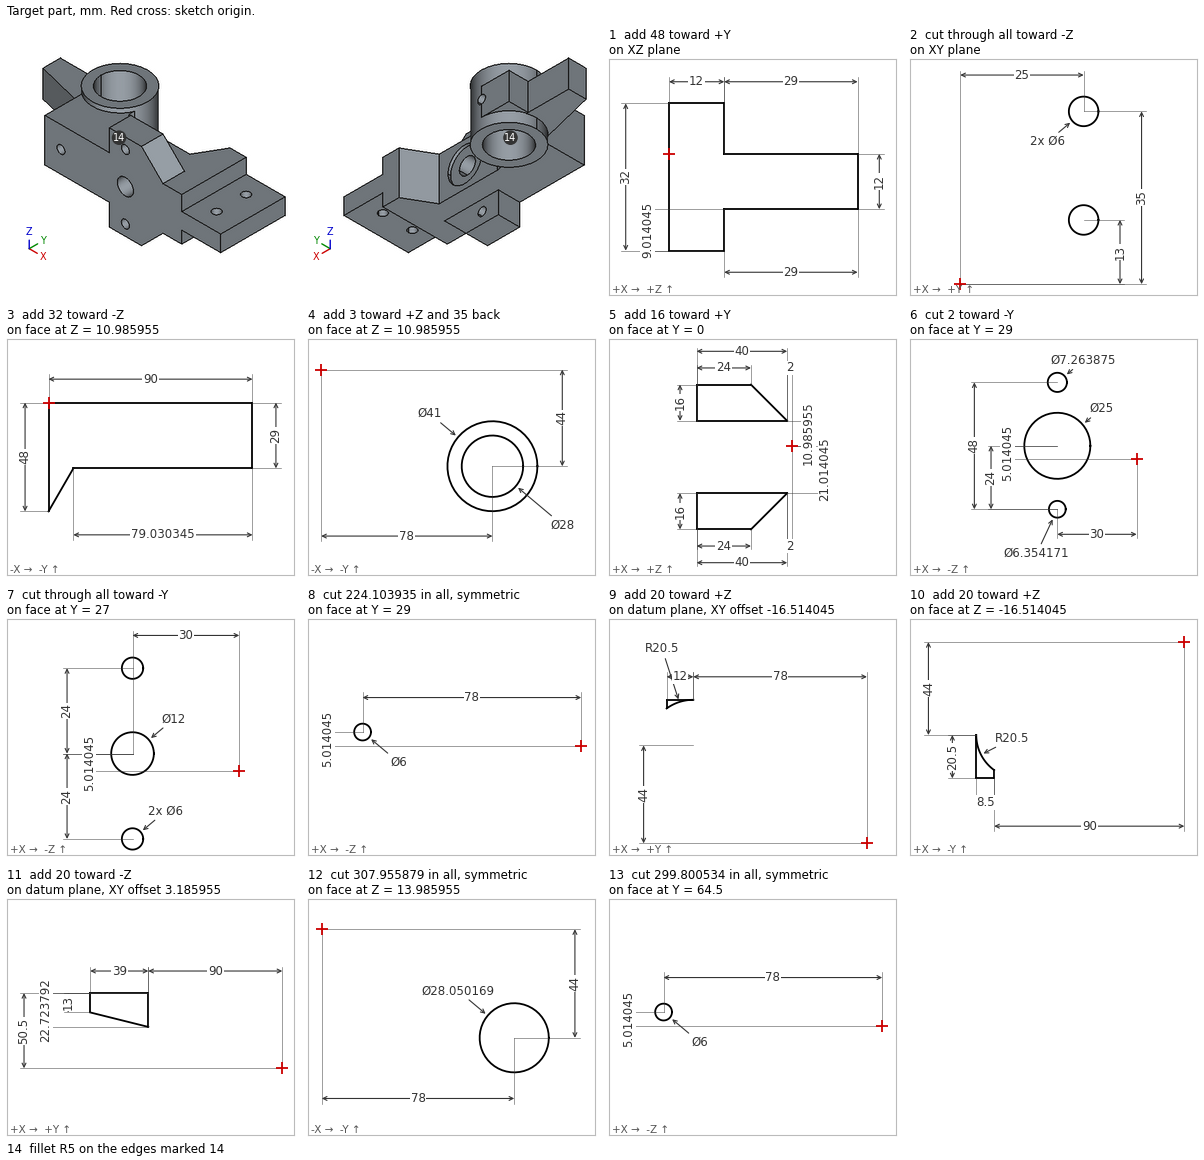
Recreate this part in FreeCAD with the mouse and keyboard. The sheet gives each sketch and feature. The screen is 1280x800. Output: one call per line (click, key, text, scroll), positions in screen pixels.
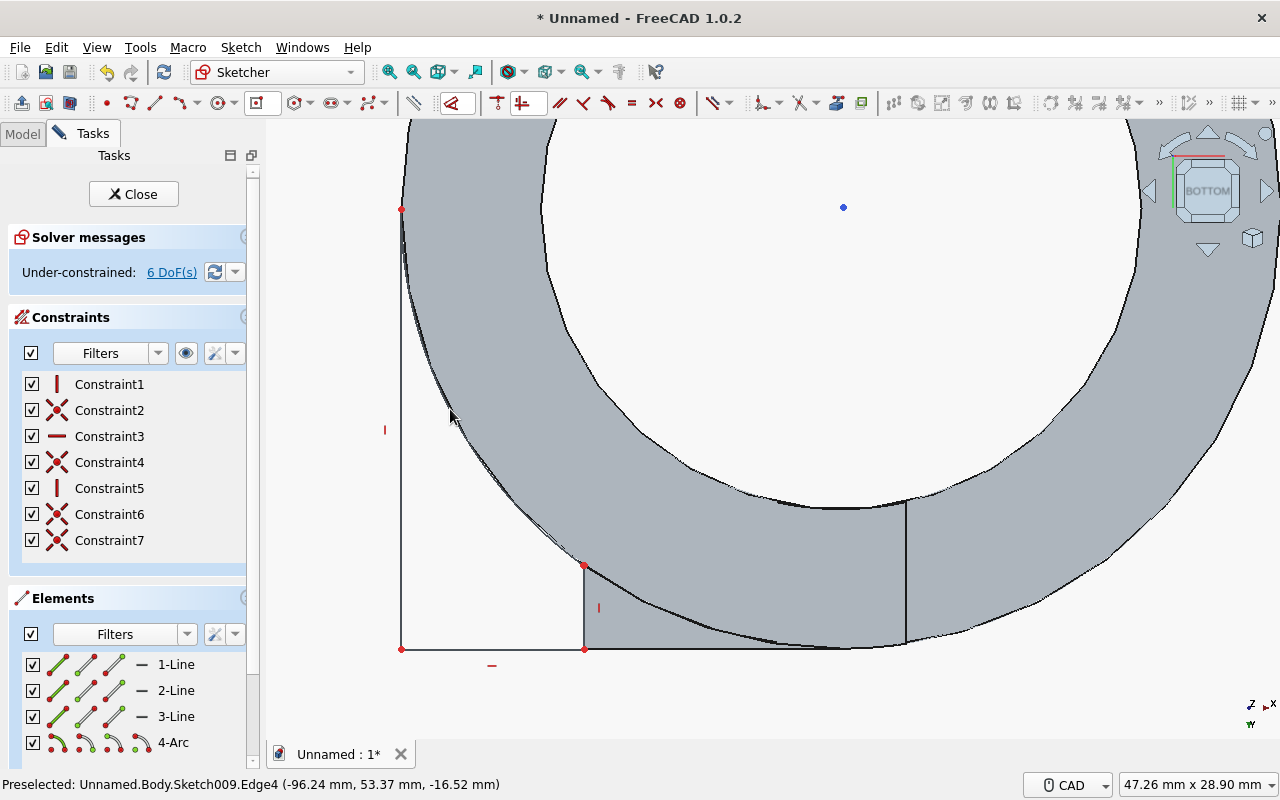
click(401, 518)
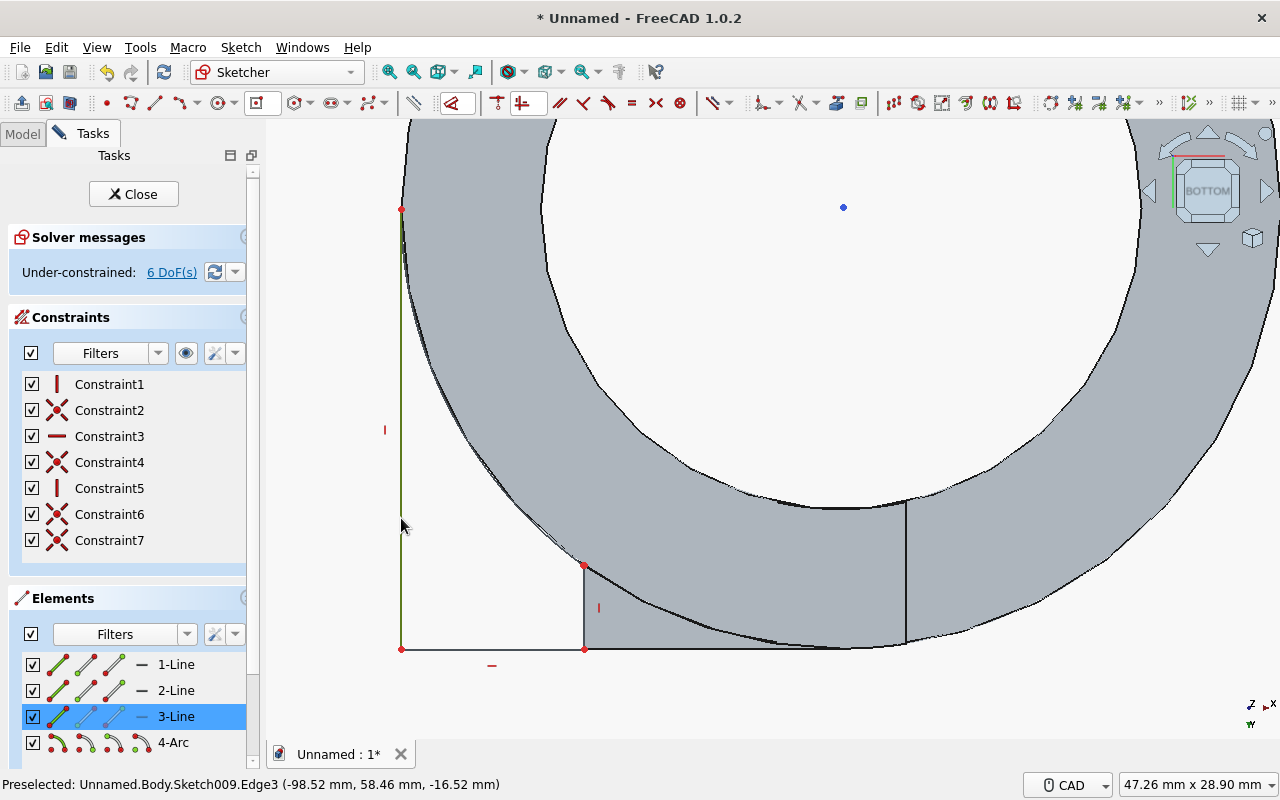
click(419, 333)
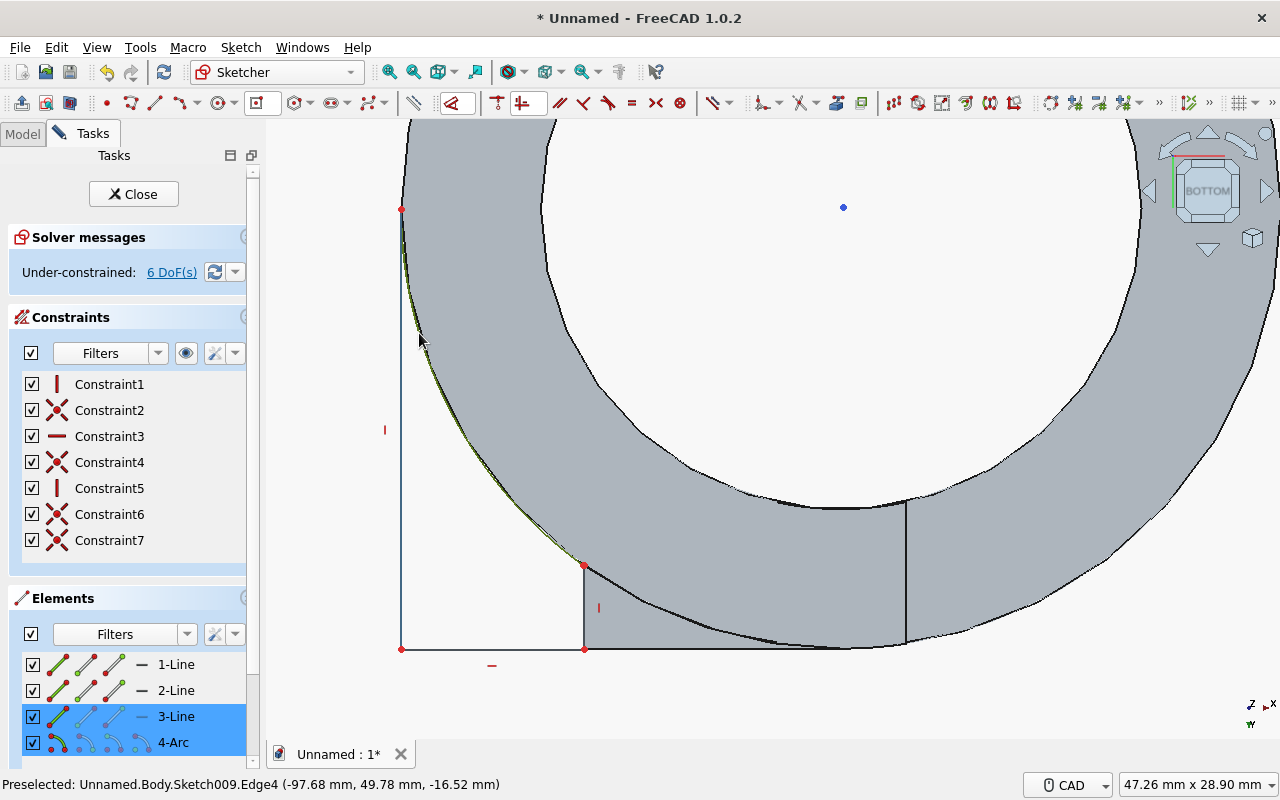
click(608, 104)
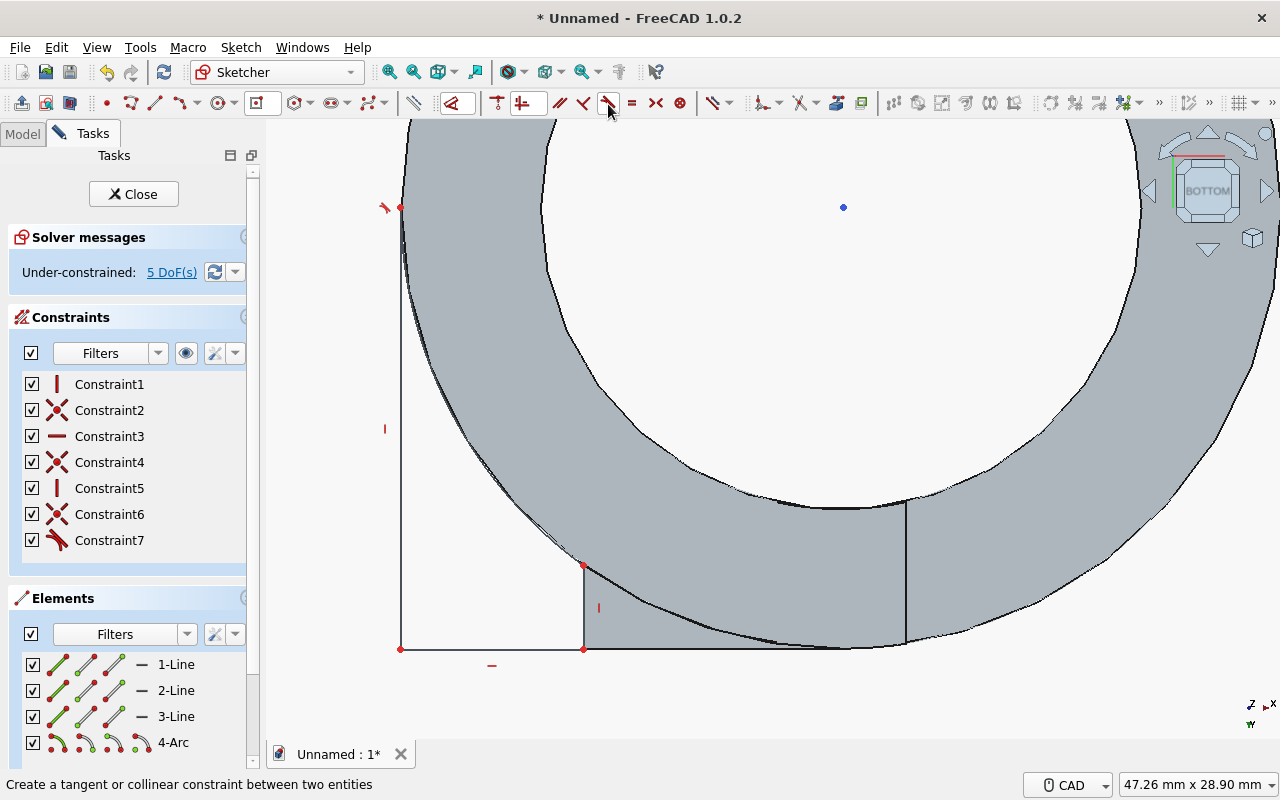
click(419, 331)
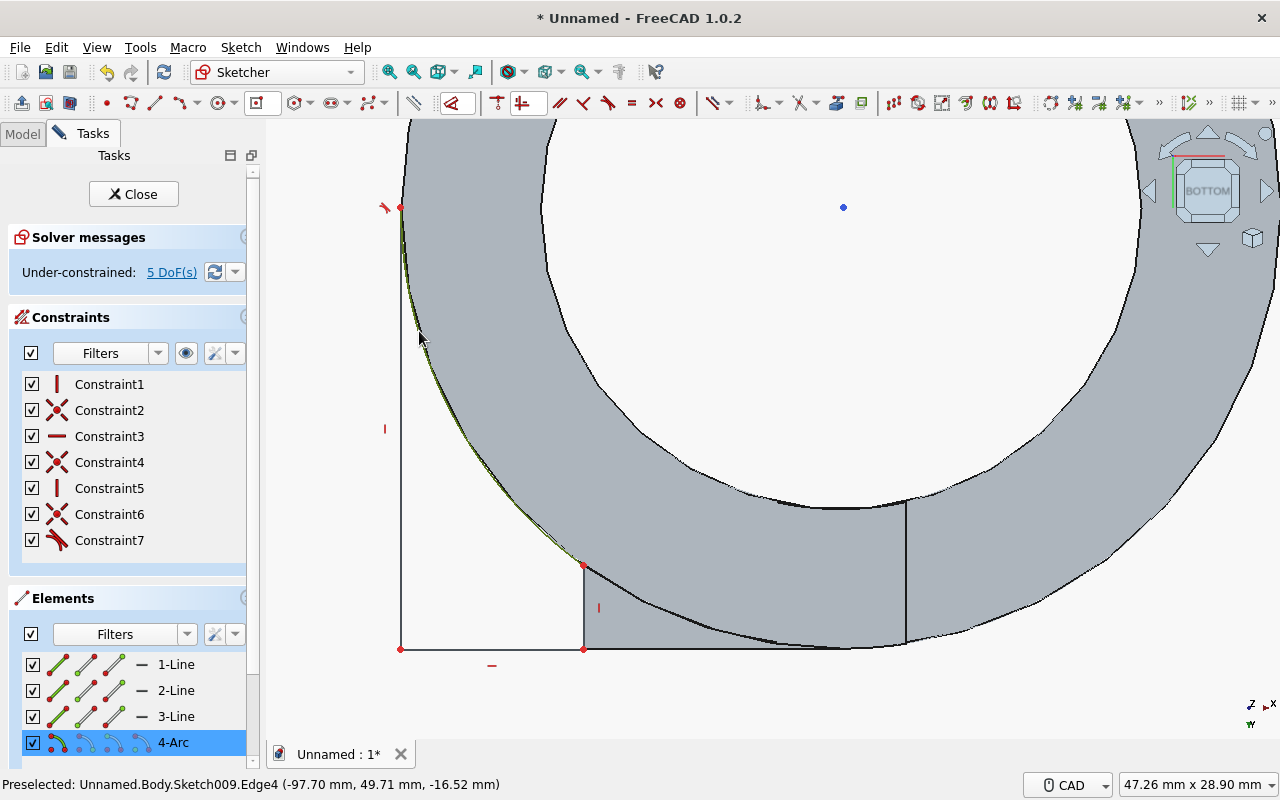
key(k)
key(r)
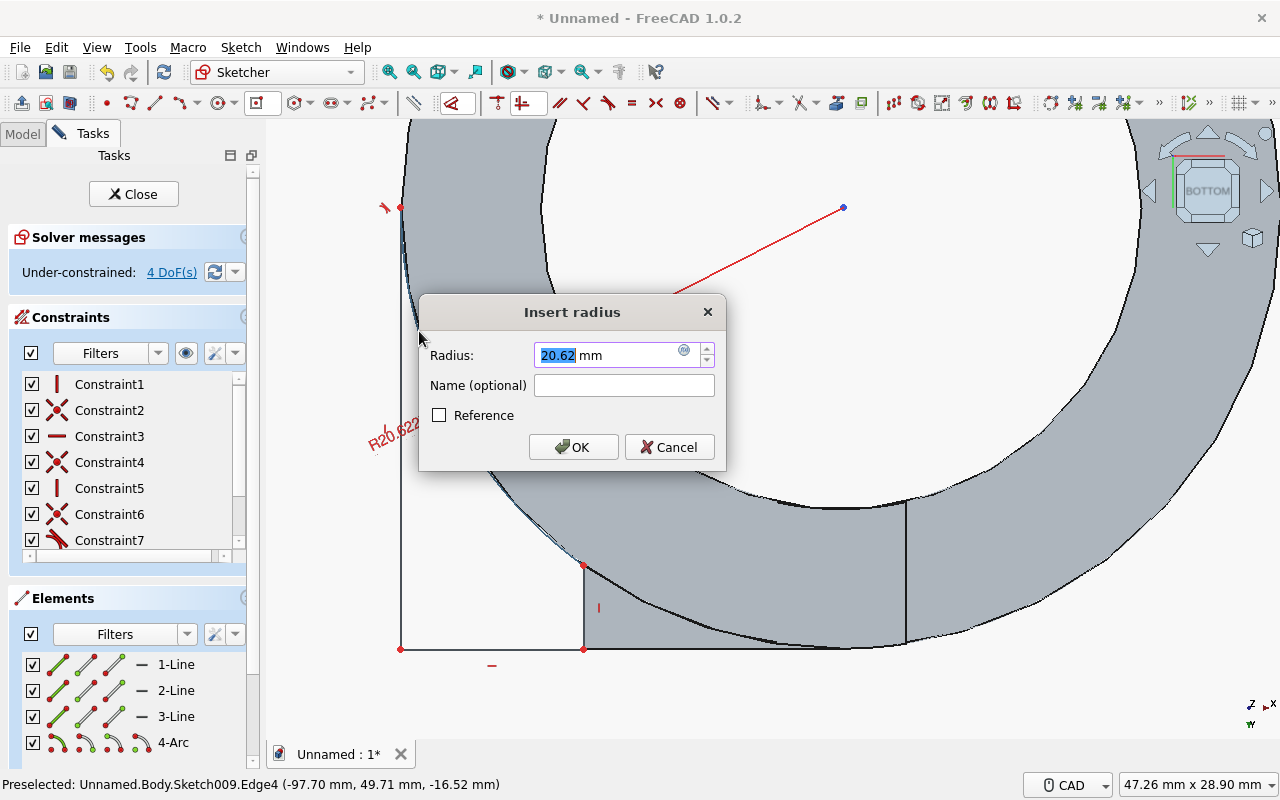
text(20.5)
key(Return)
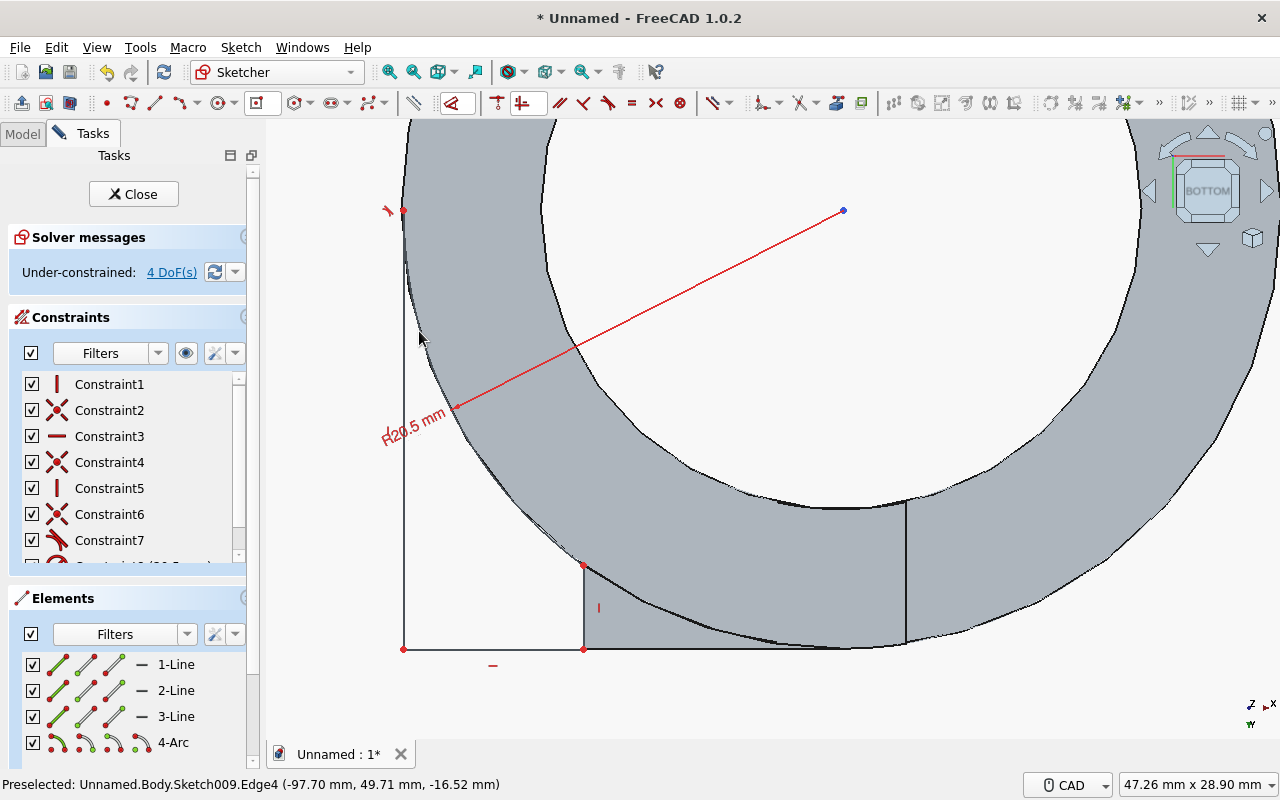
click(530, 650)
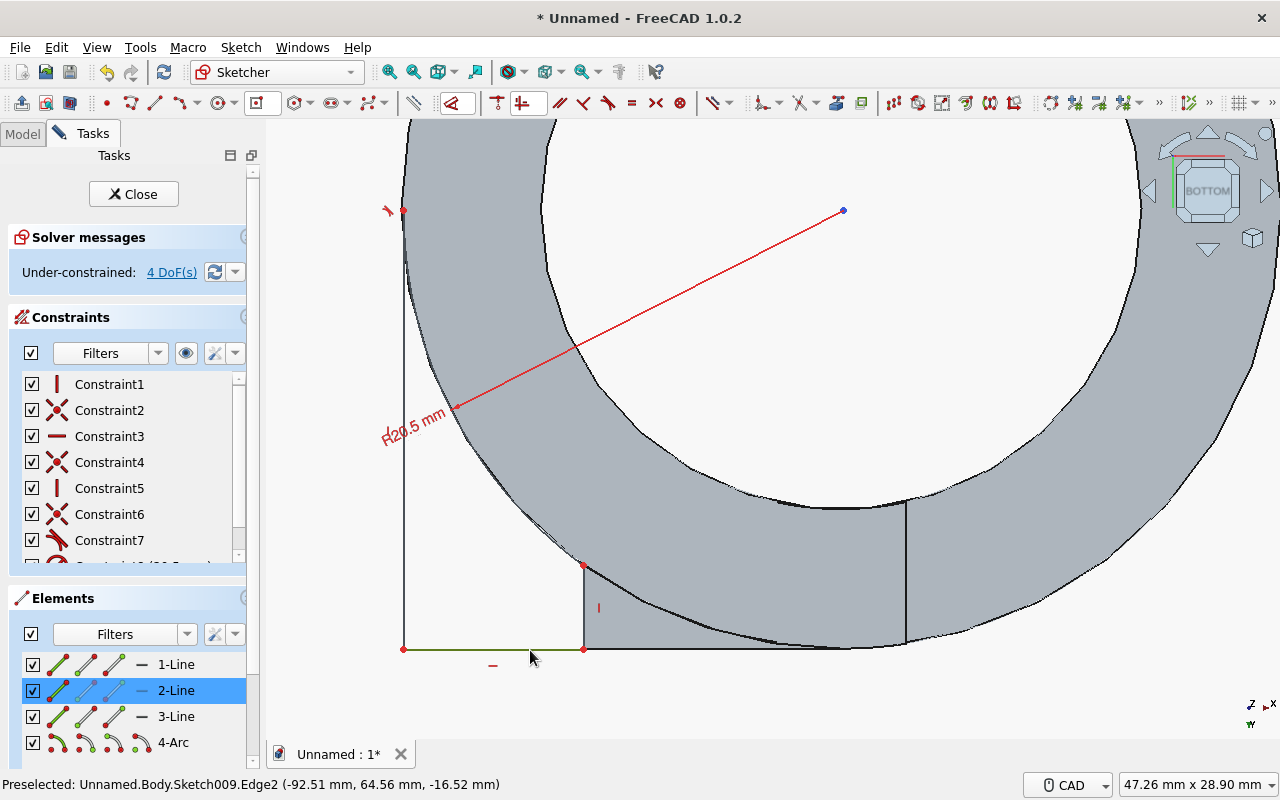
key(l)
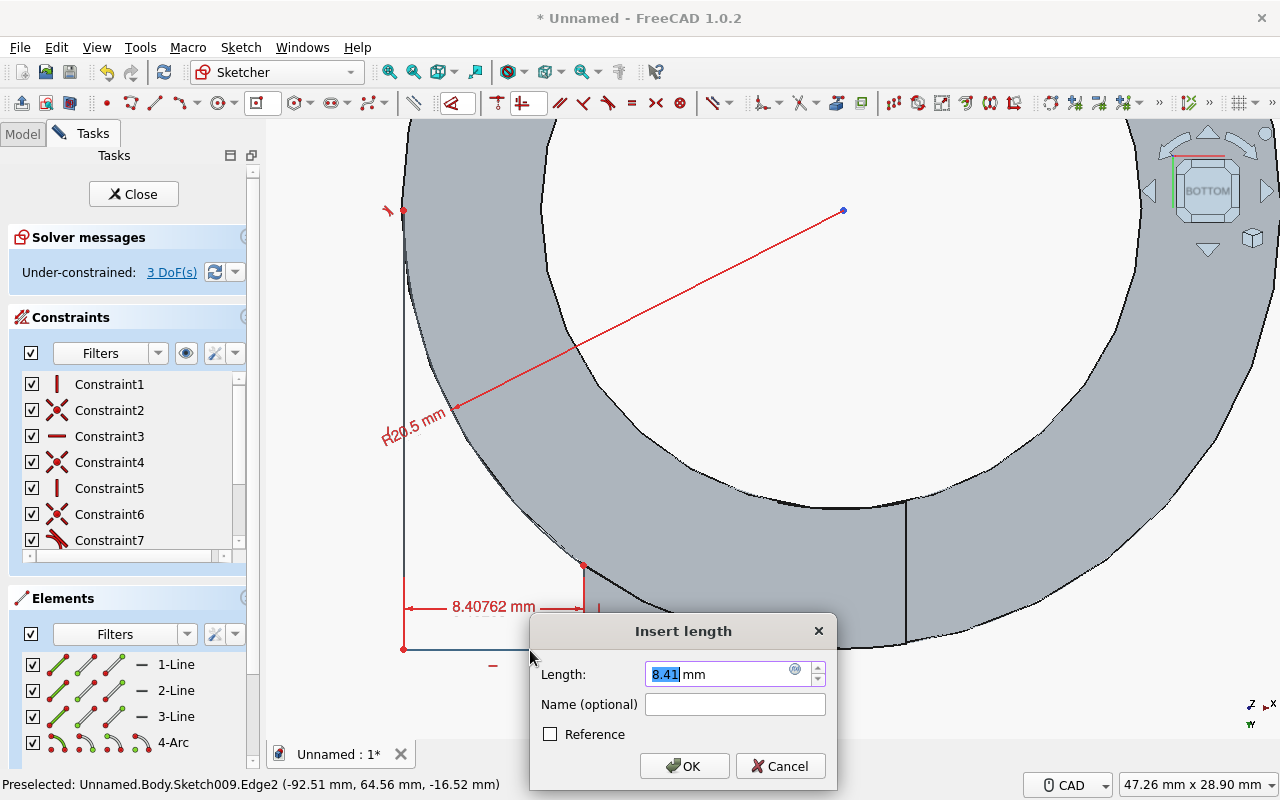
text(8.5)
key(Return)